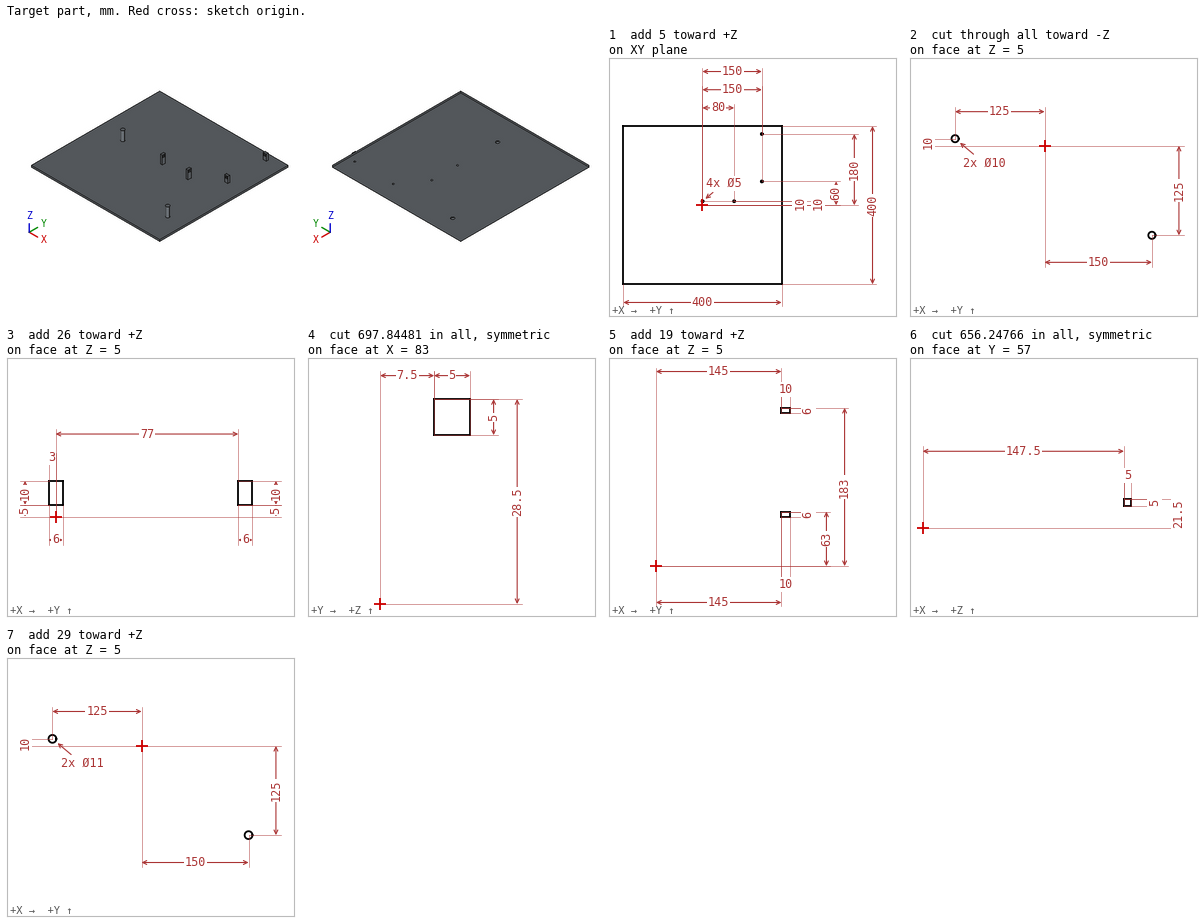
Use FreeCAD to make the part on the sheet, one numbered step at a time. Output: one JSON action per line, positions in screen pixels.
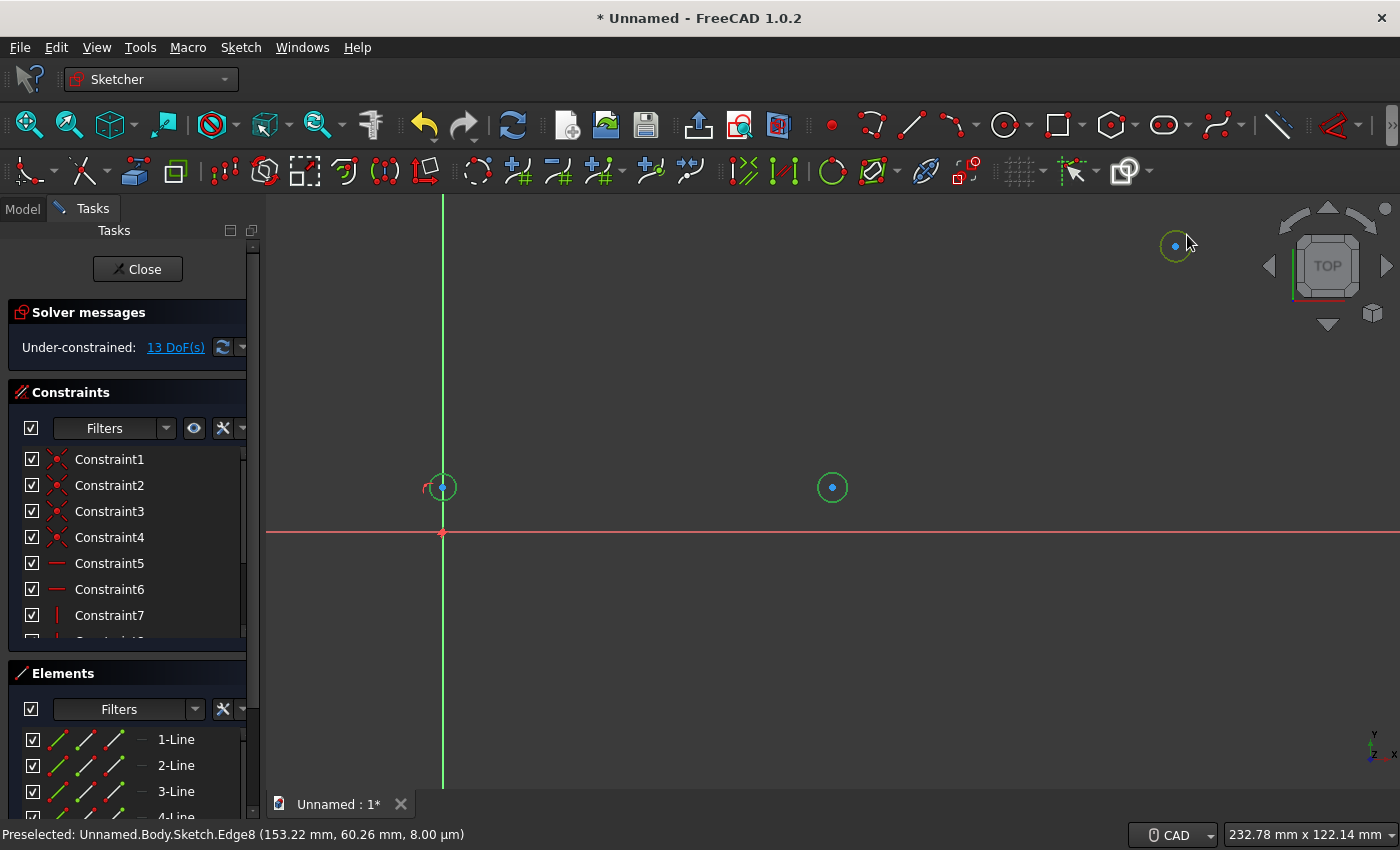
{"action": "scroll", "coordinate": [846, 481], "scroll_direction": "down", "scroll_amount": 8}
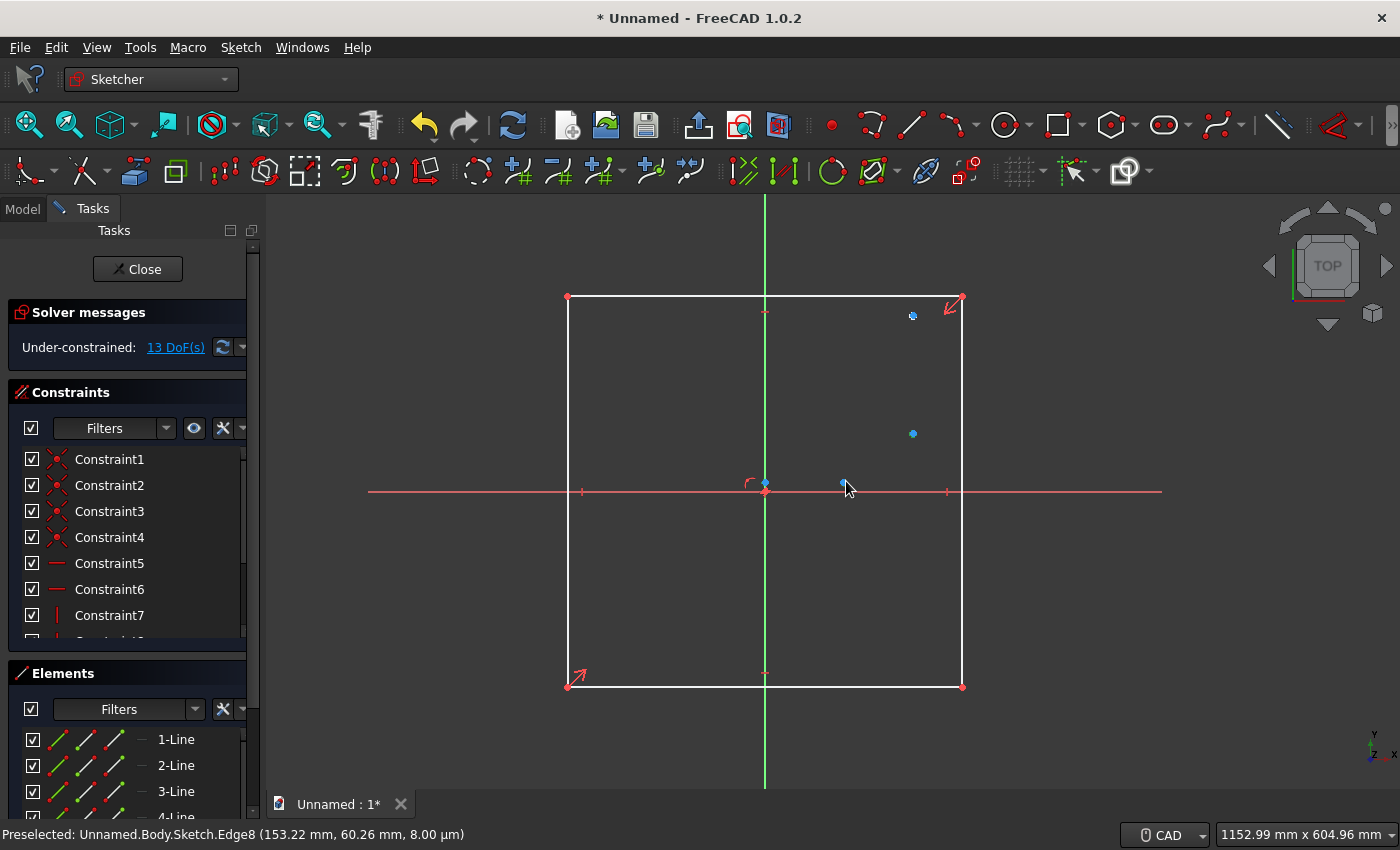
{"action": "scroll", "coordinate": [915, 314], "scroll_direction": "up", "scroll_amount": 8}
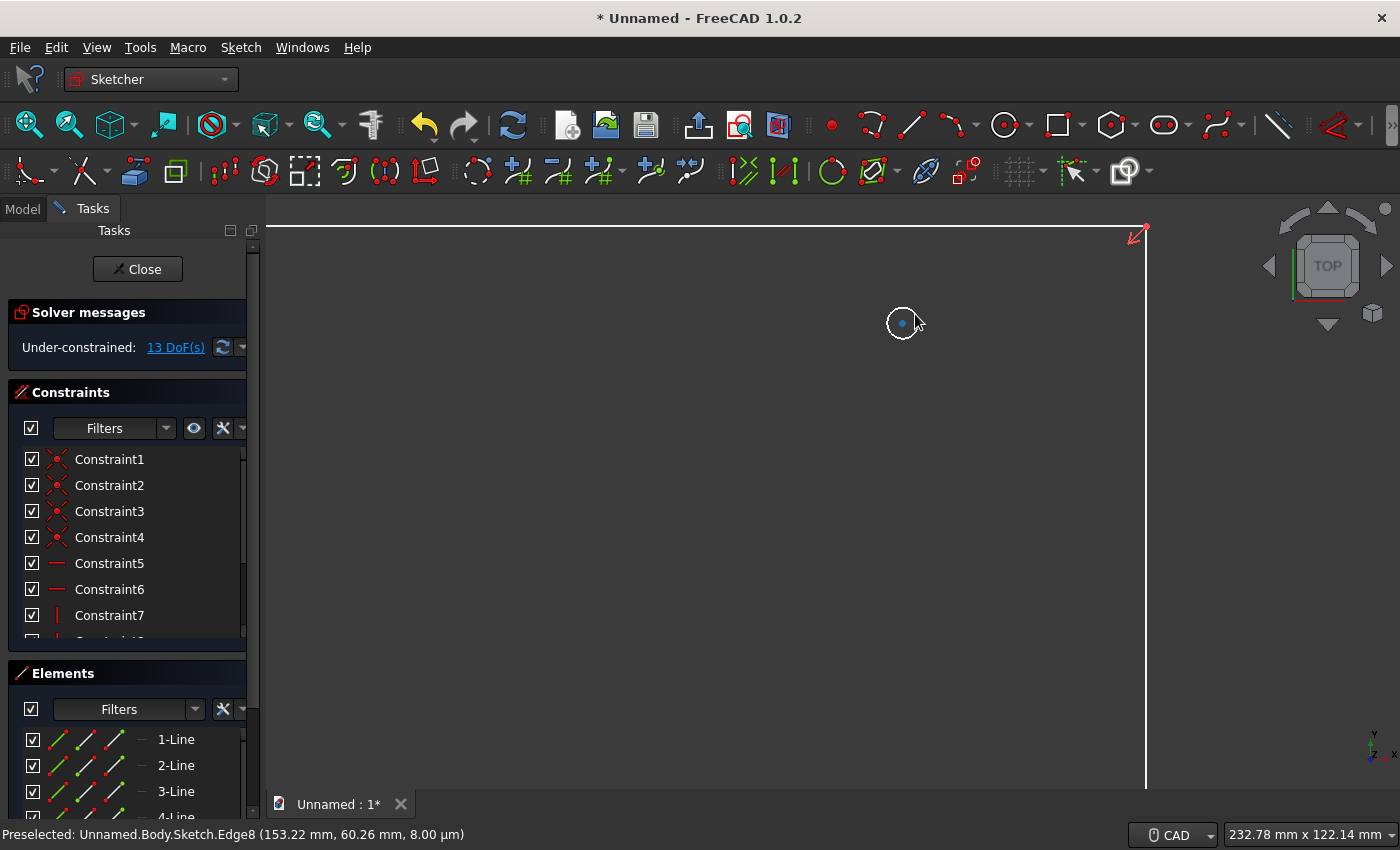
{"action": "left_click", "coordinate": [914, 312]}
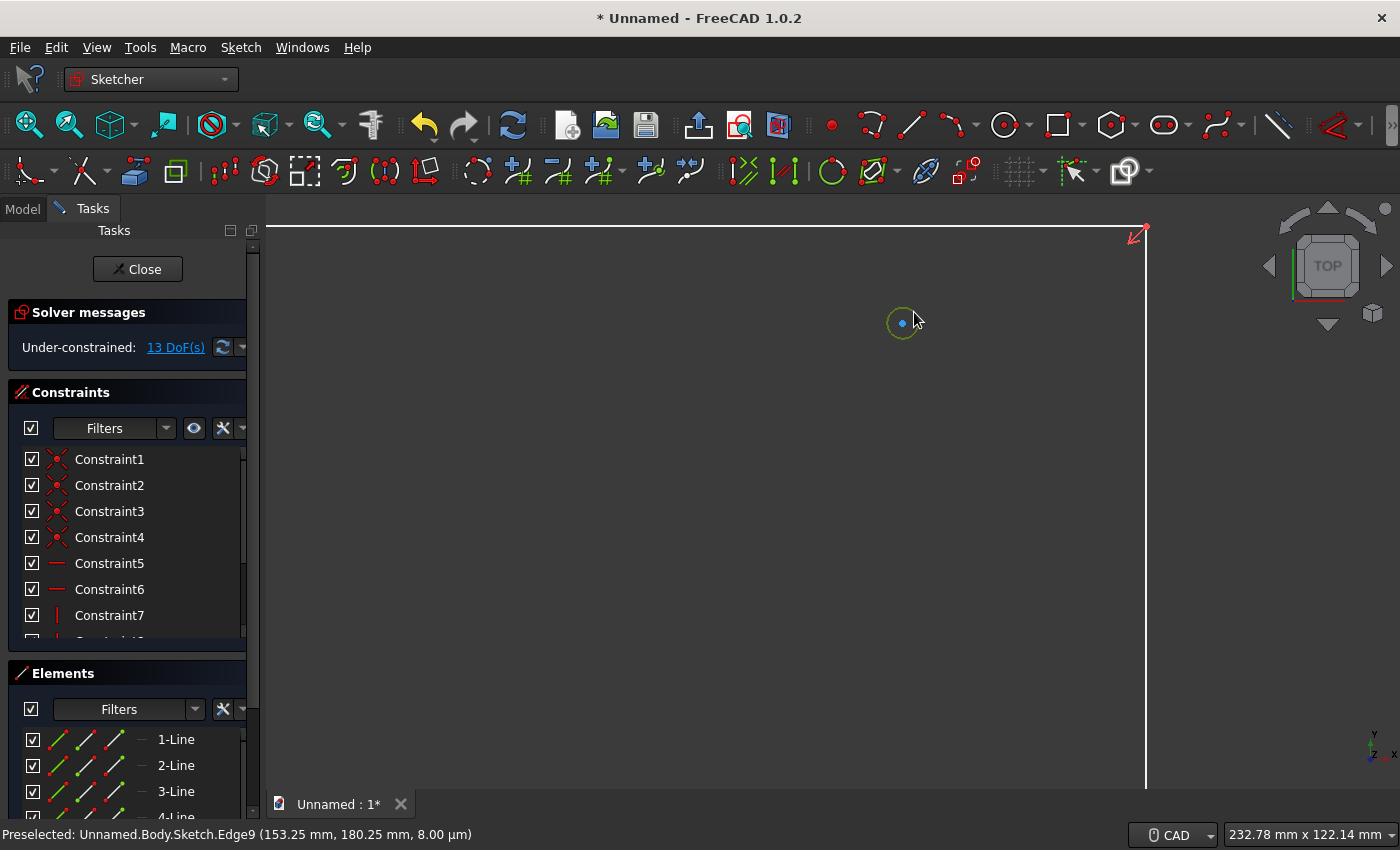
{"action": "key", "text": "e"}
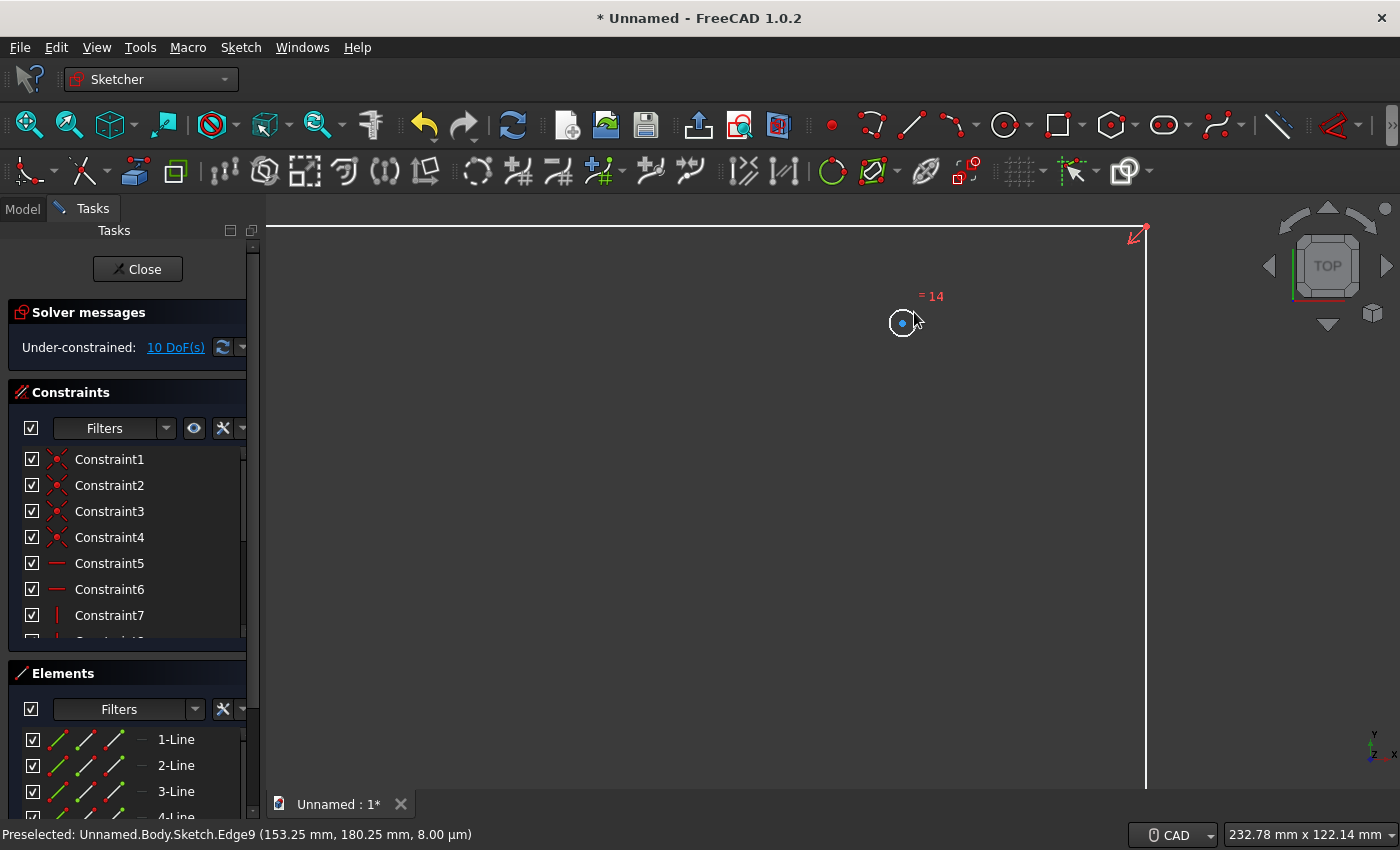
{"action": "scroll", "coordinate": [915, 314], "scroll_direction": "down", "scroll_amount": 8}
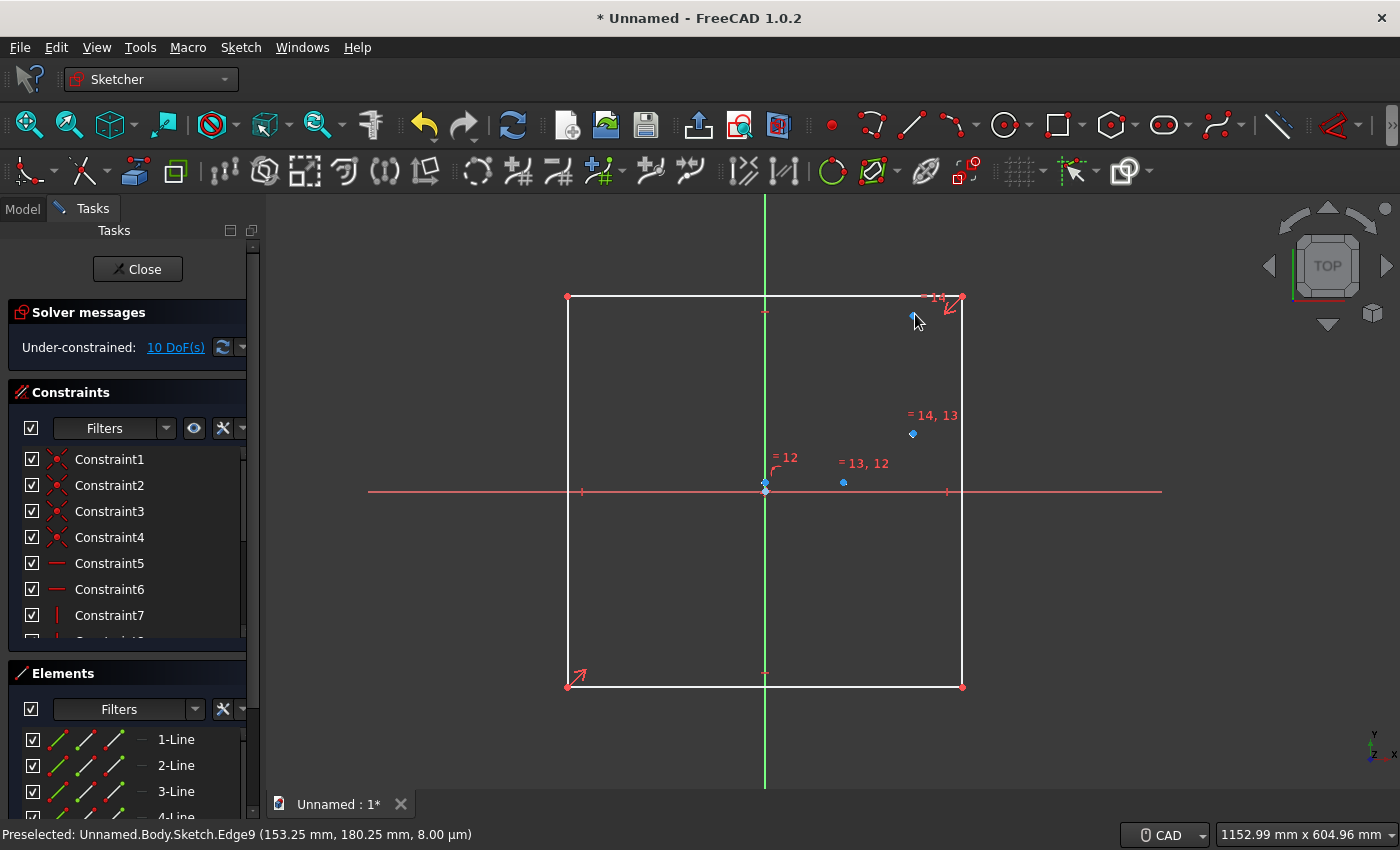
{"action": "scroll", "coordinate": [767, 481], "scroll_direction": "up", "scroll_amount": 11}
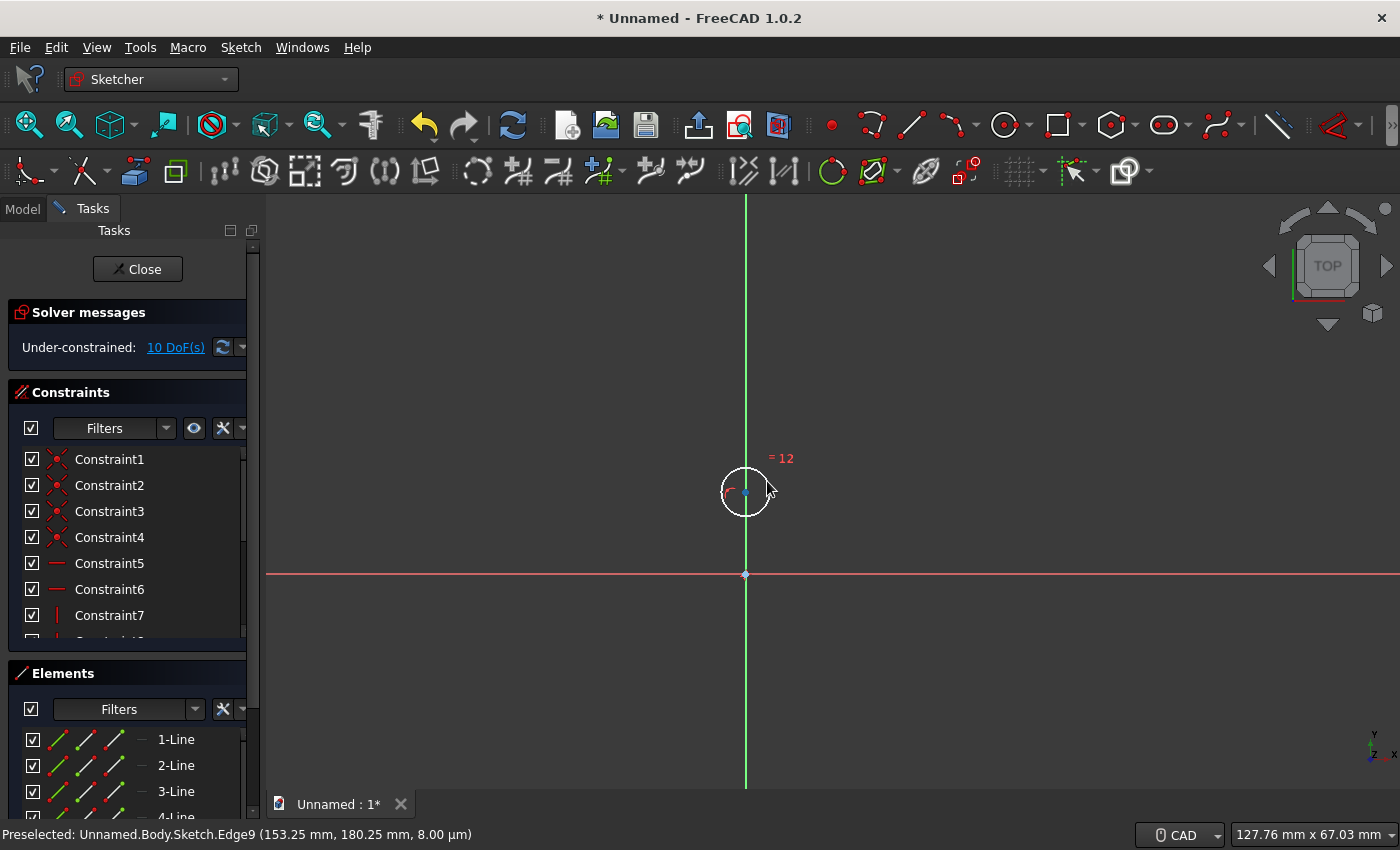
{"action": "left_click", "coordinate": [763, 475]}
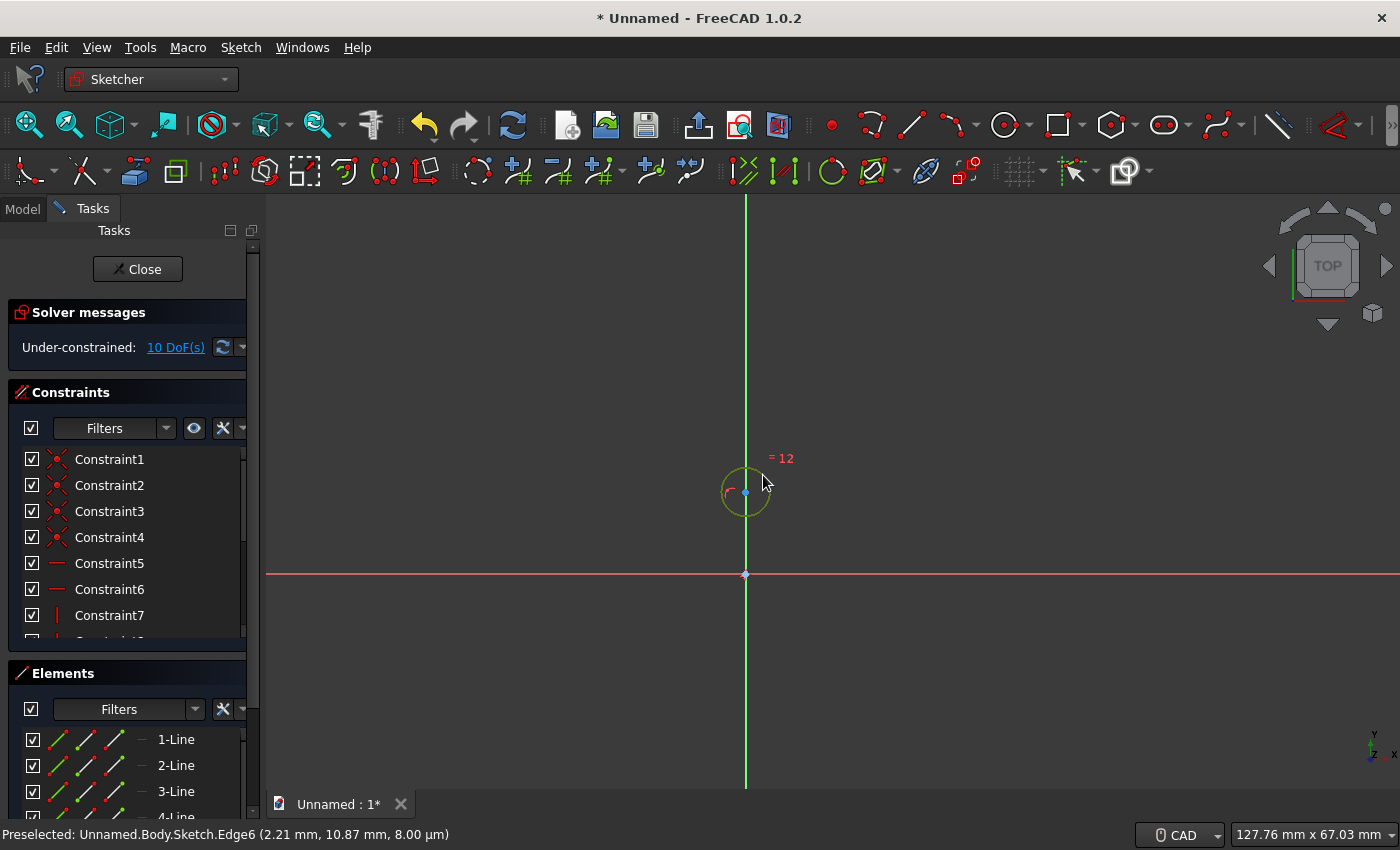
{"action": "key", "text": "k o"}